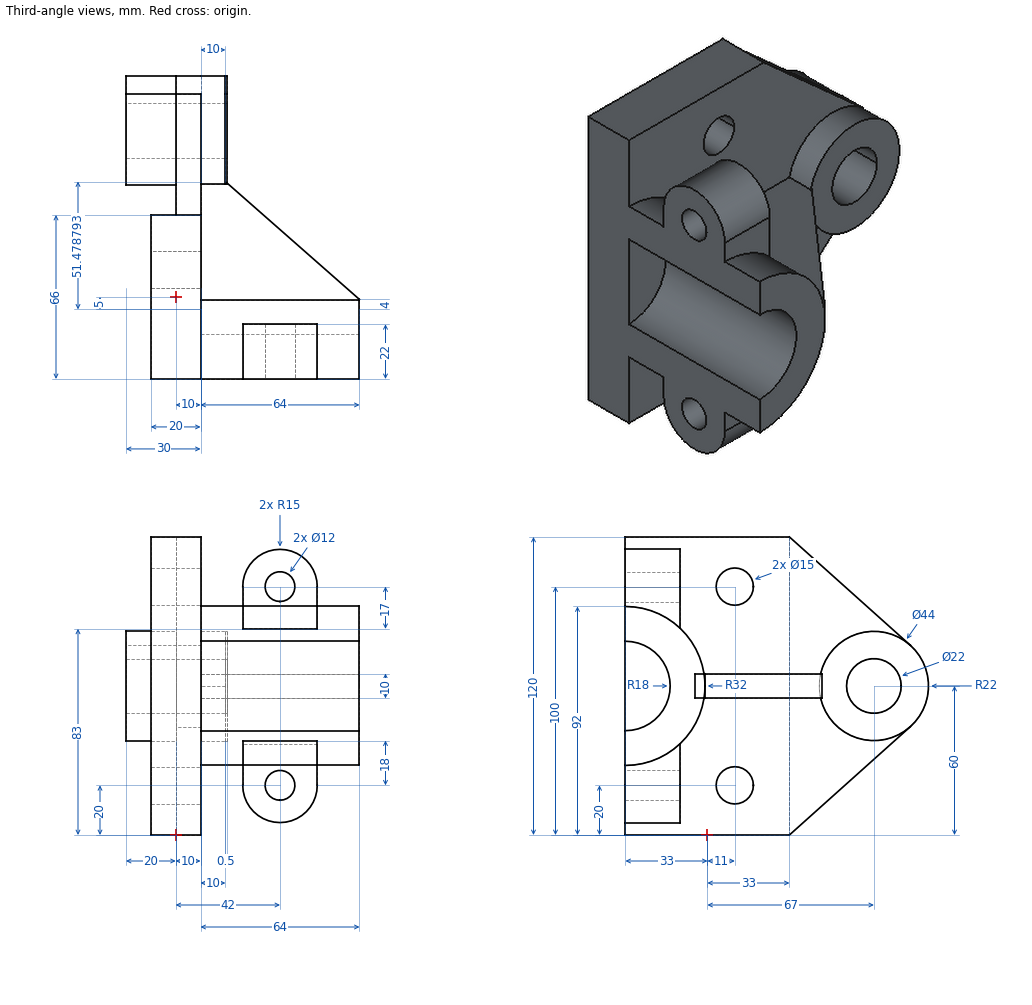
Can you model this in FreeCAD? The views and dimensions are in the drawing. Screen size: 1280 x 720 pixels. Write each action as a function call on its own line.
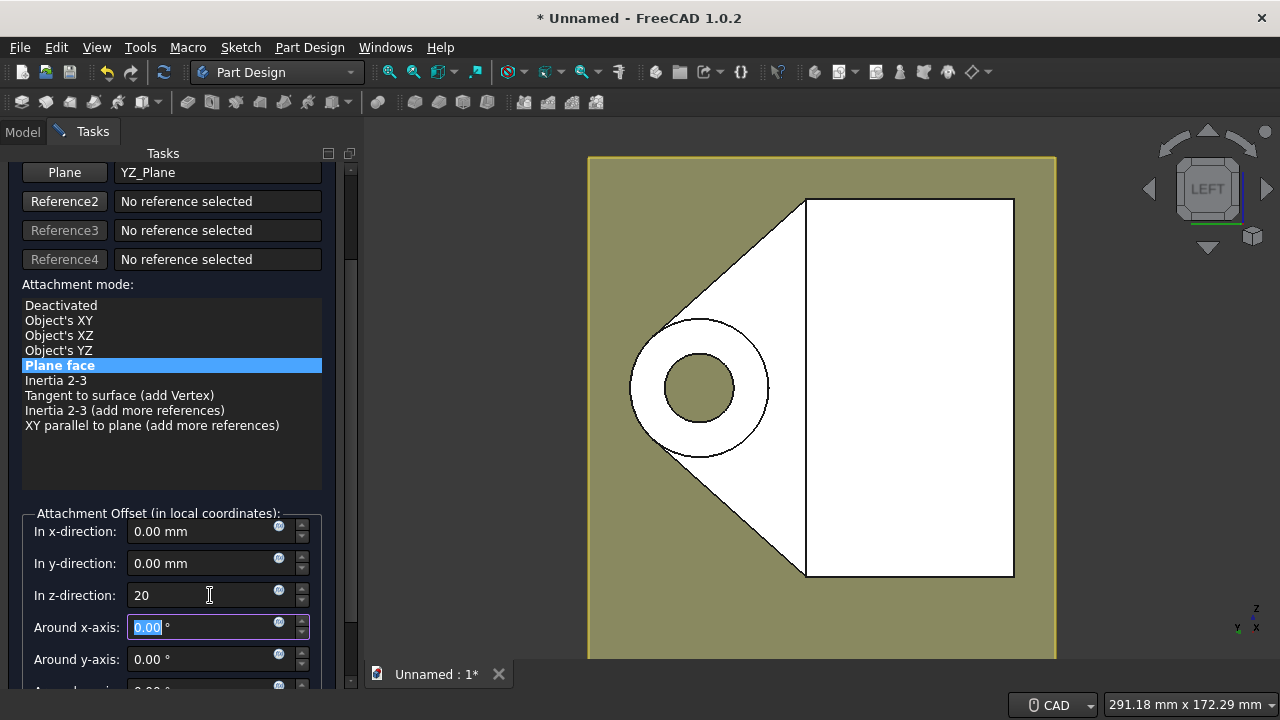
scroll(351, 426, up, 3)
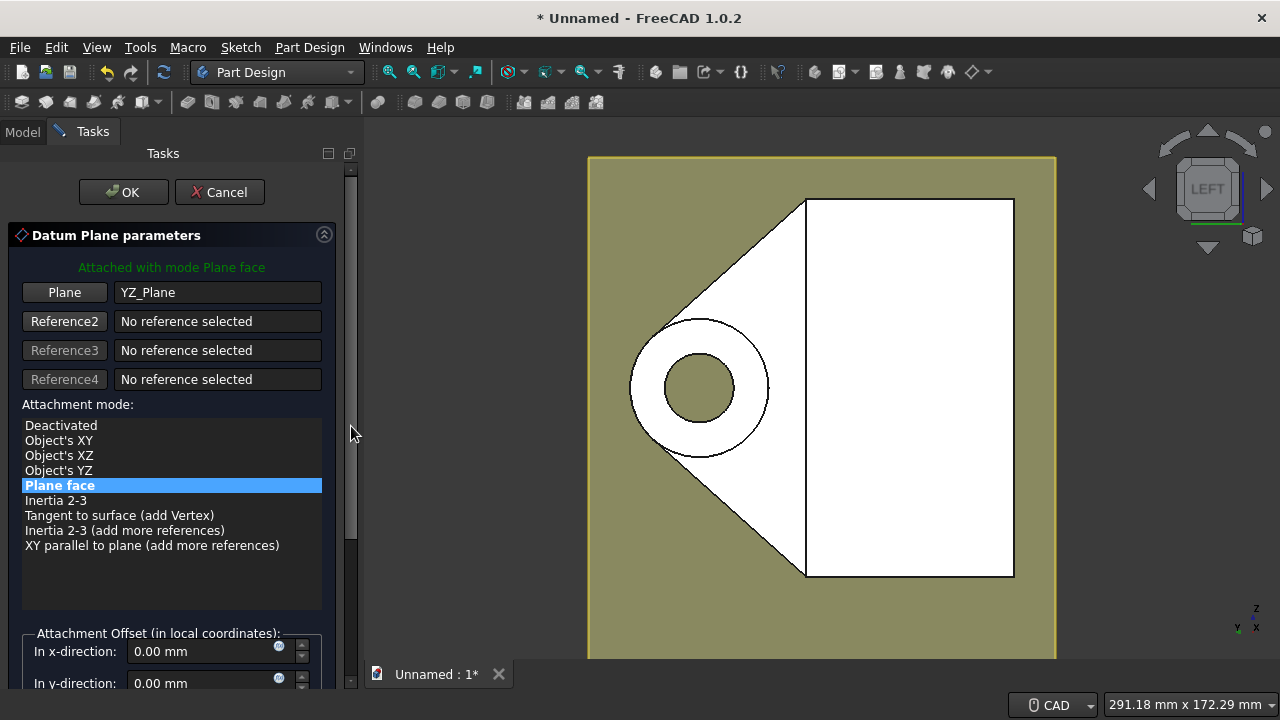
click(124, 192)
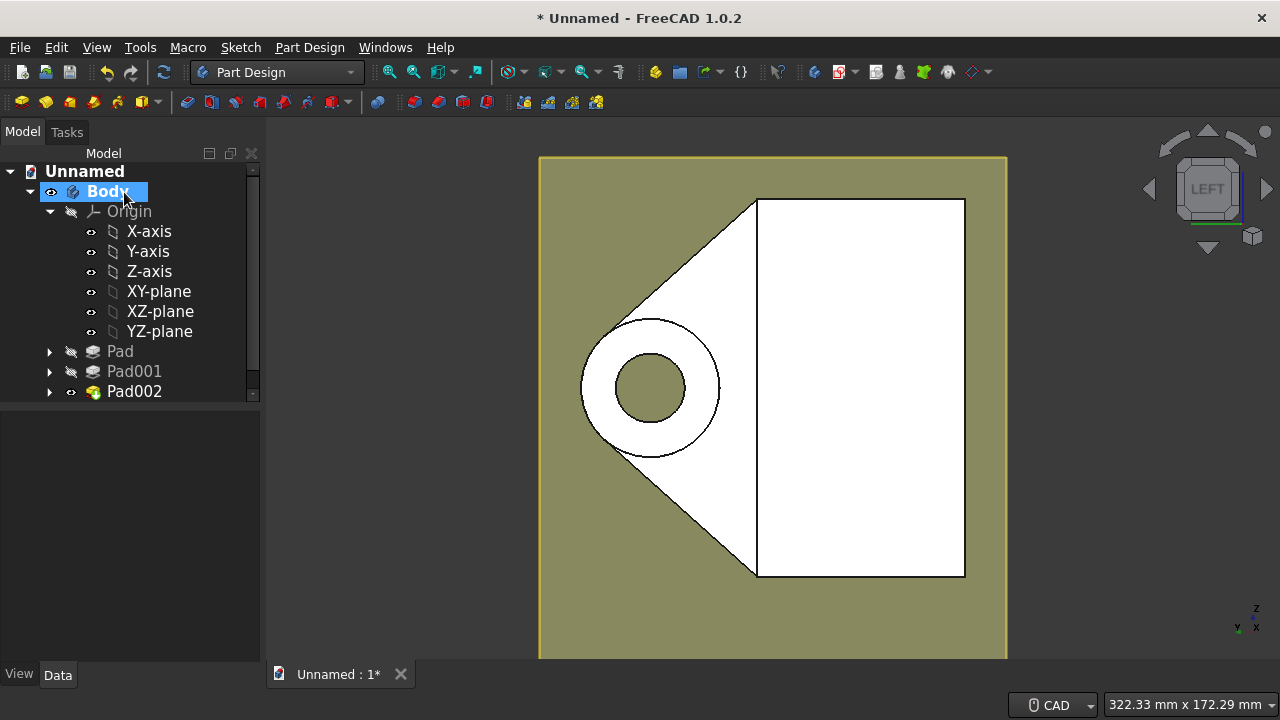
scroll(100, 287, down, 3)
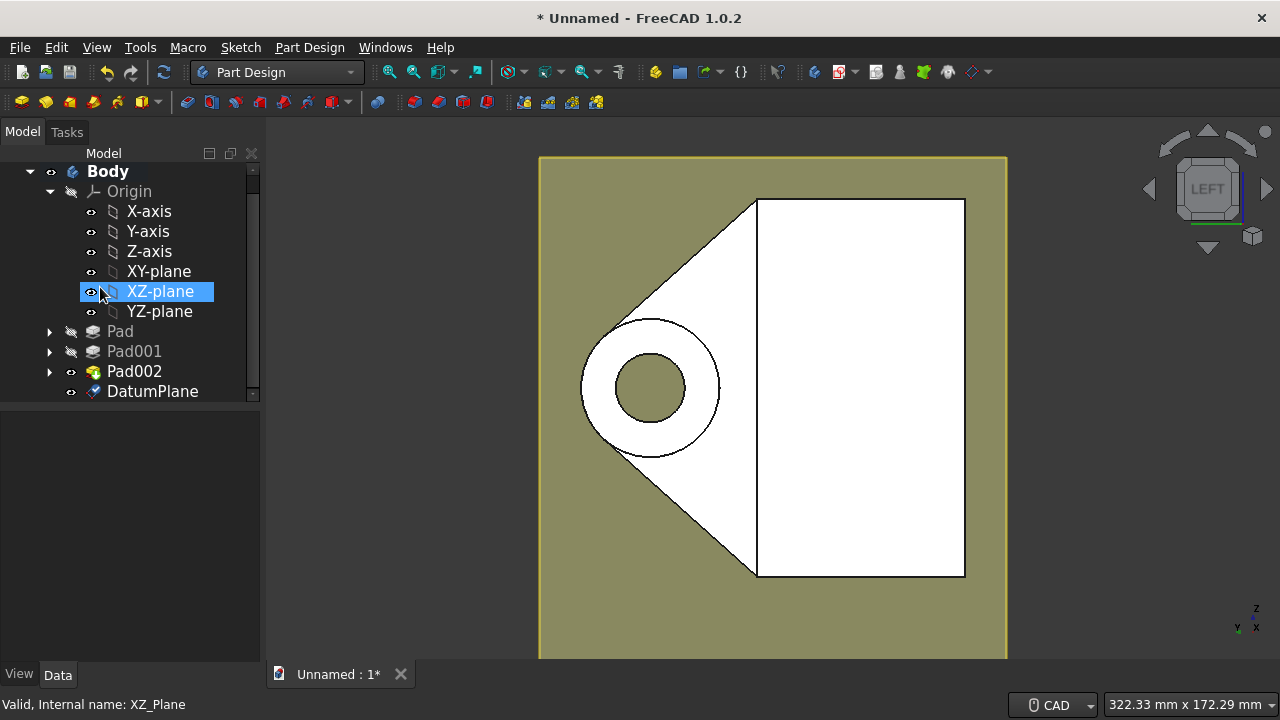
click(116, 392)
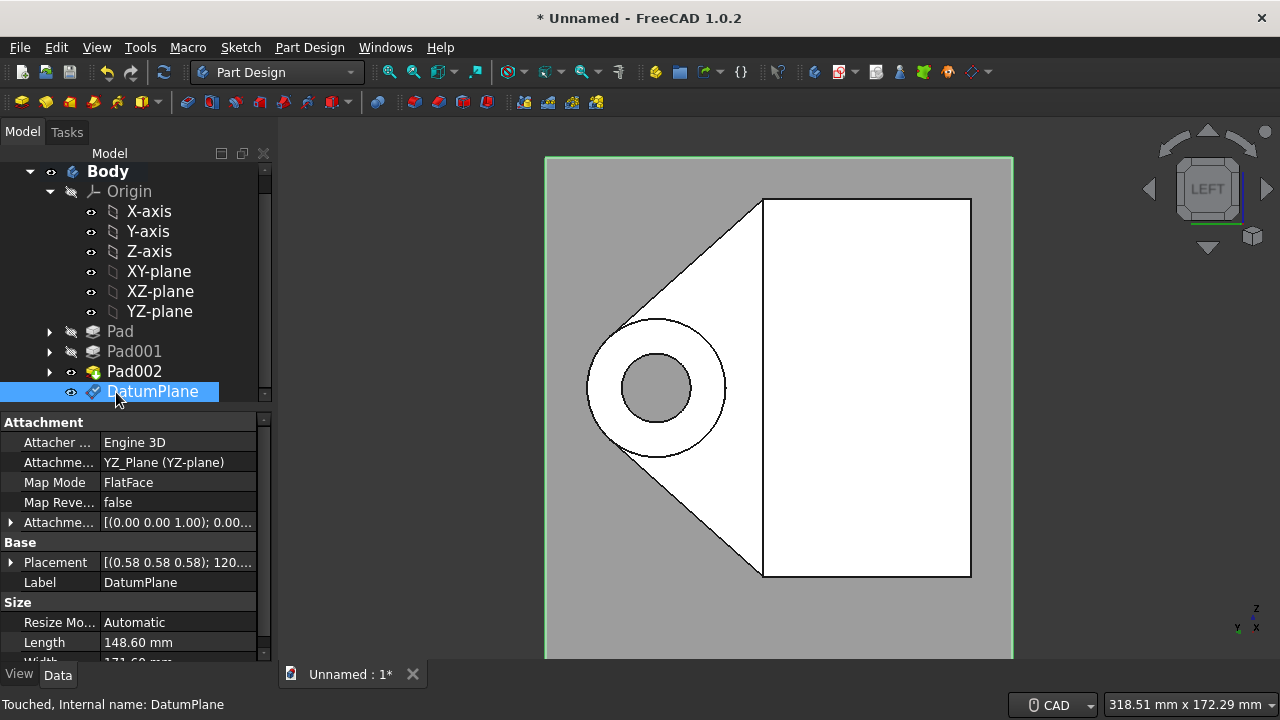
click(840, 72)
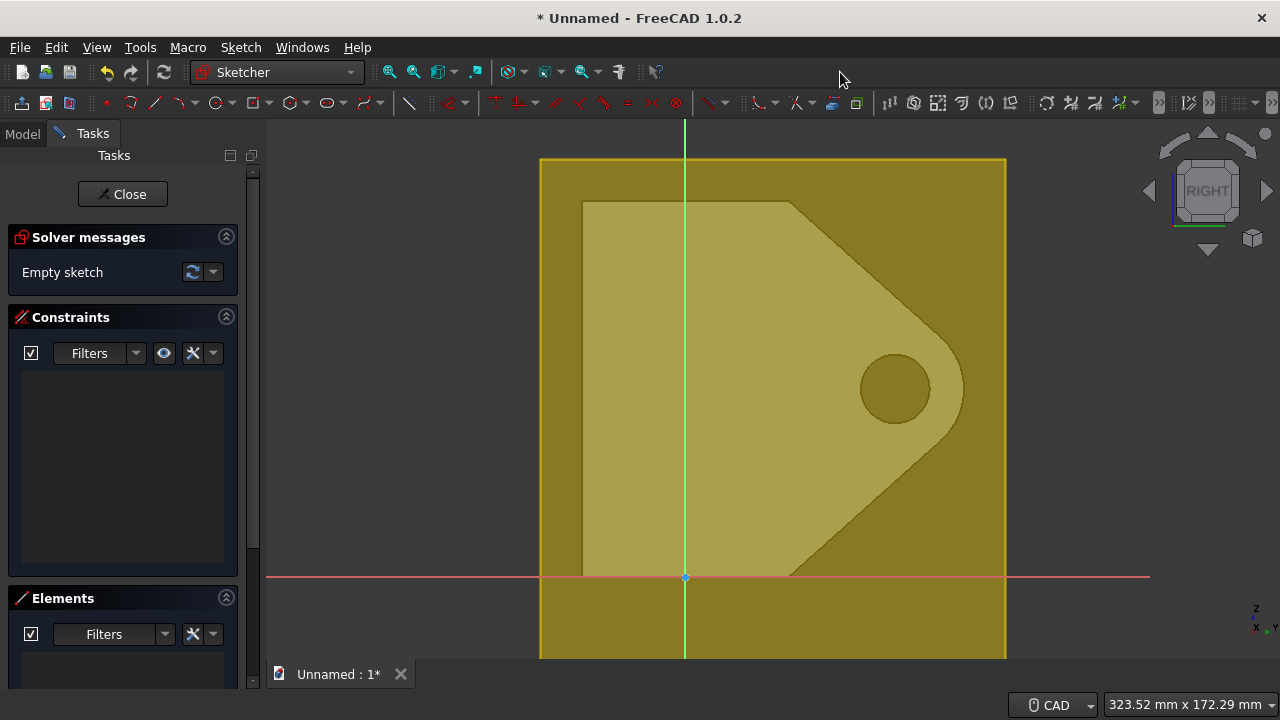
click(216, 104)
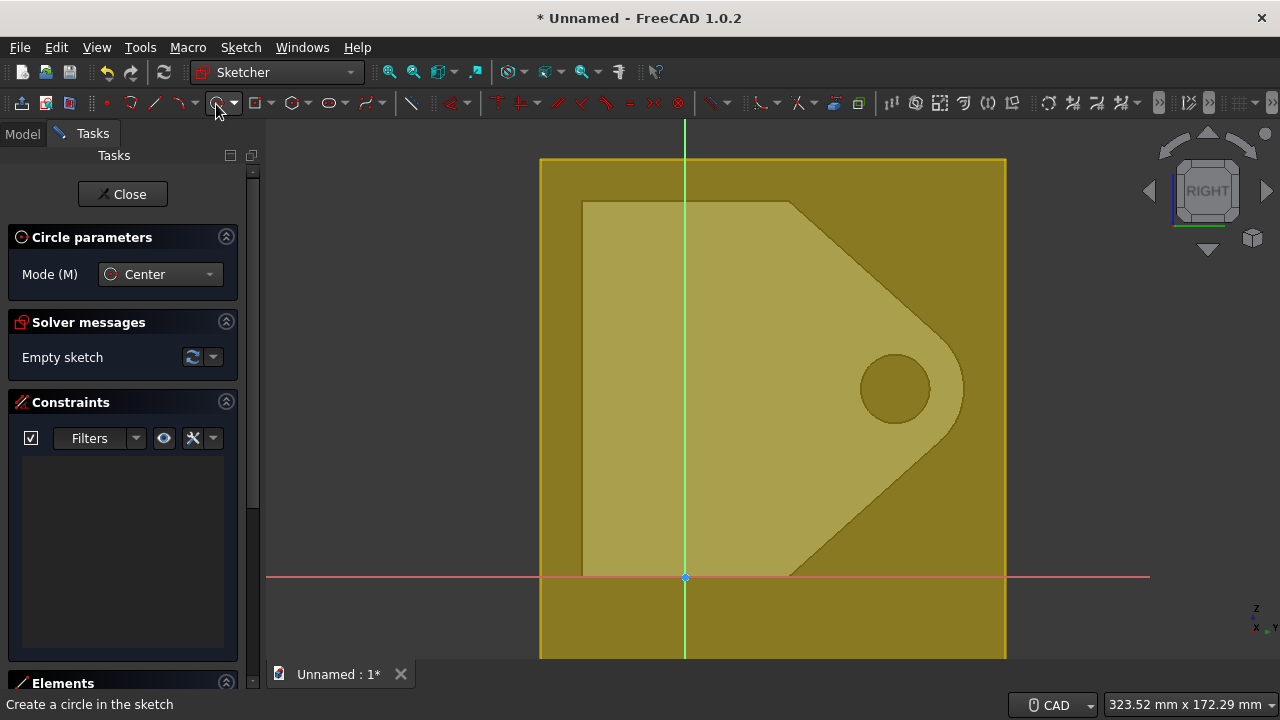
click(895, 389)
click(944, 340)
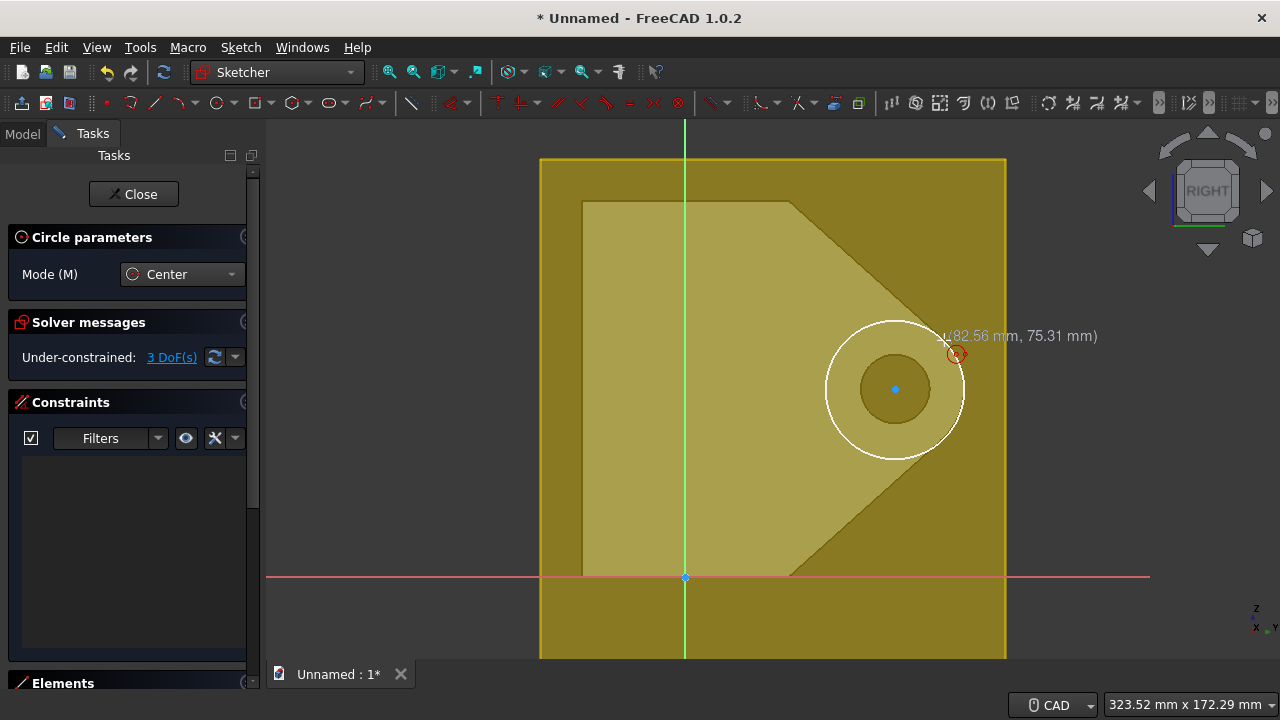
click(895, 390)
click(920, 365)
key(Escape)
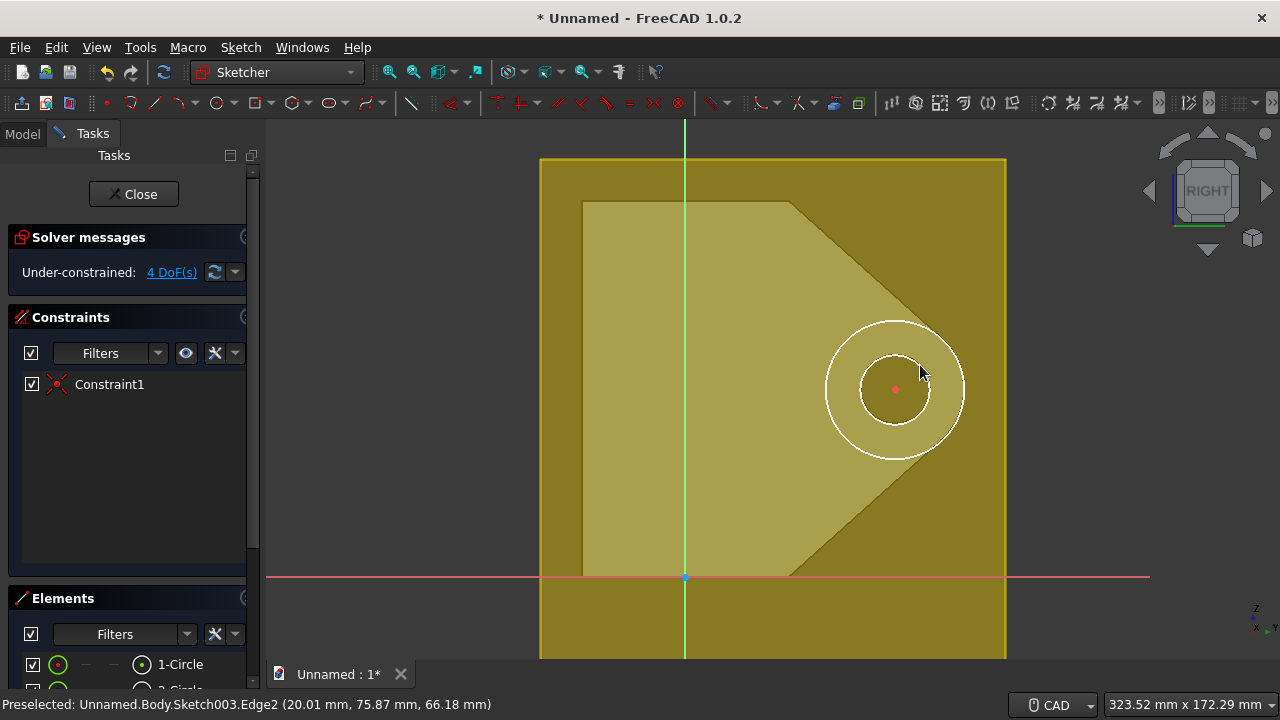
click(450, 104)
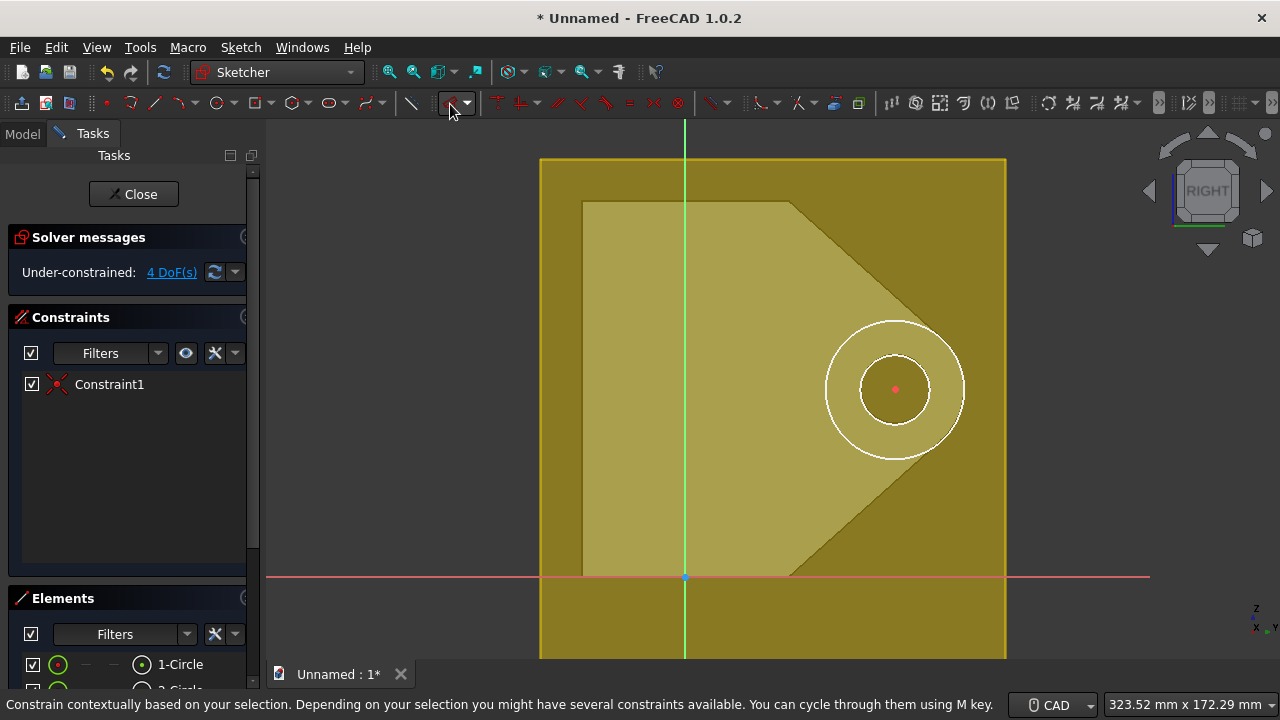
click(944, 341)
click(967, 318)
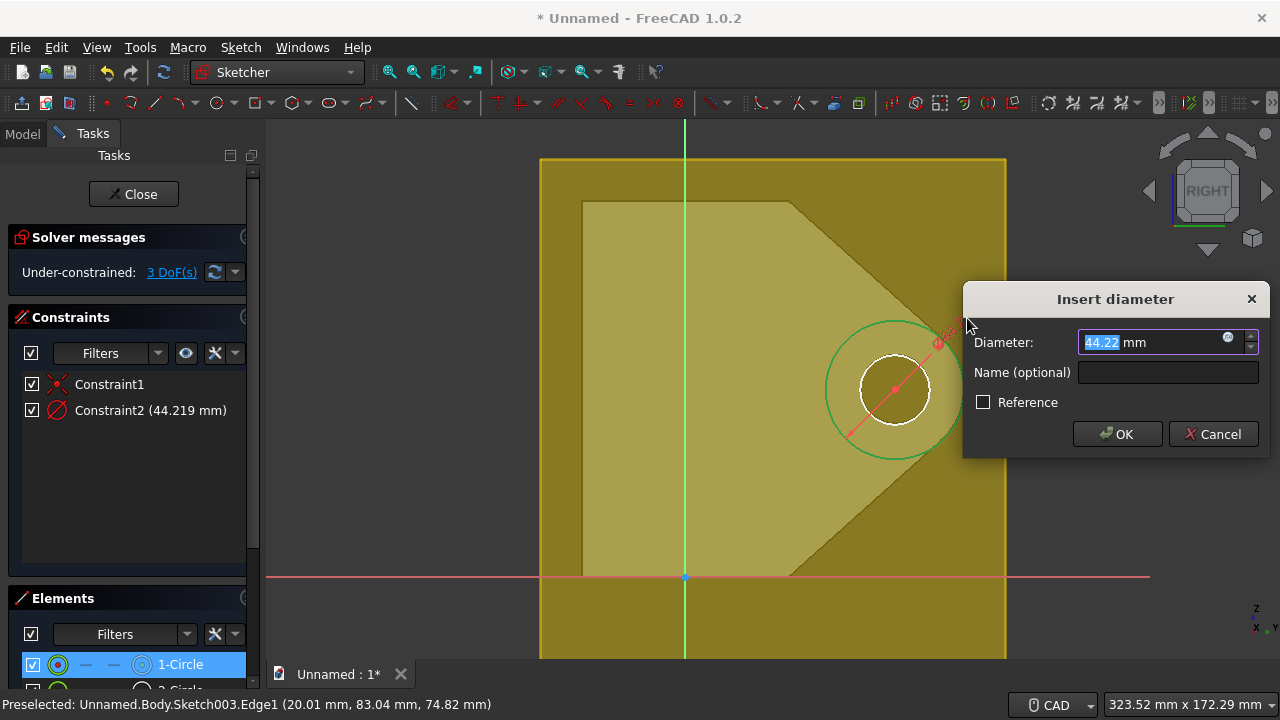
text(44)
key(Return)